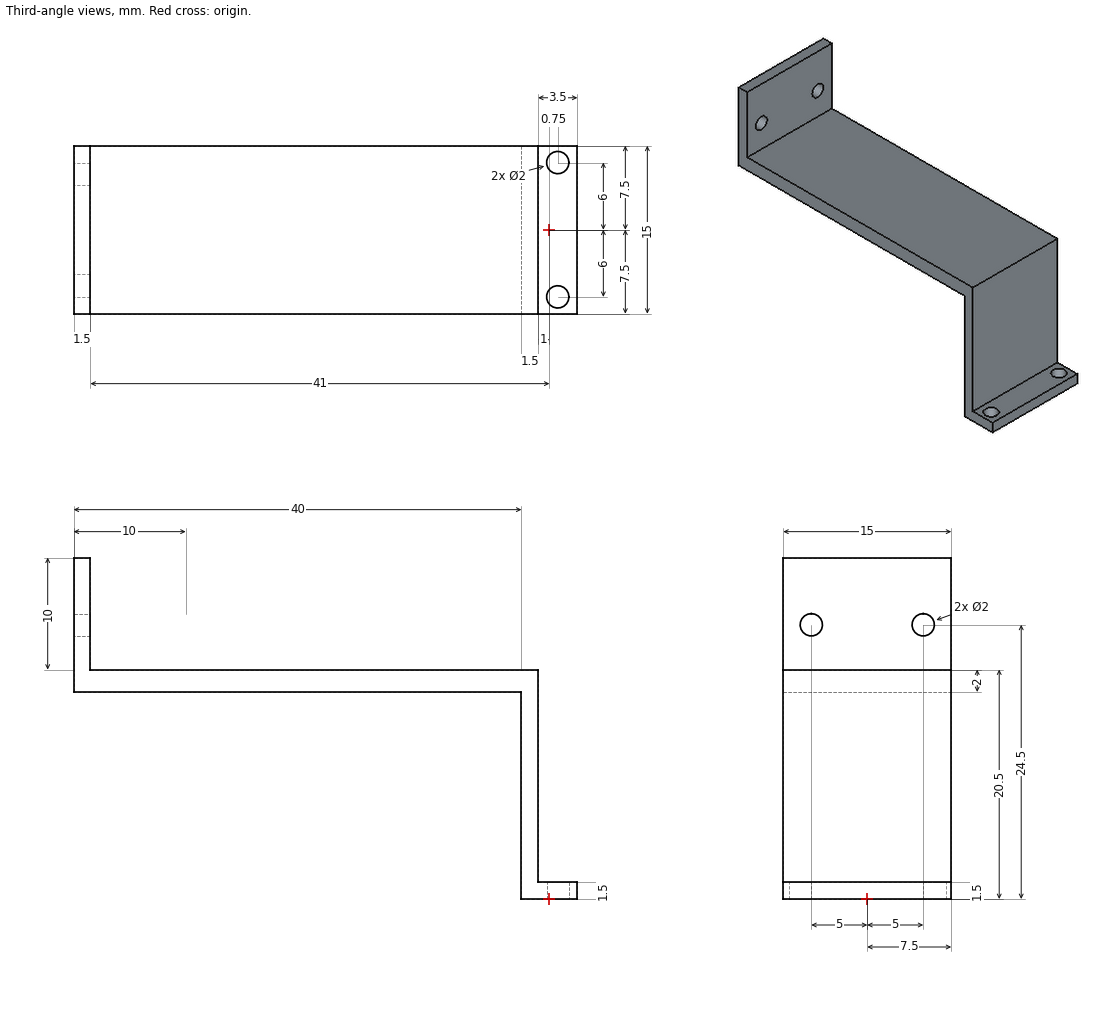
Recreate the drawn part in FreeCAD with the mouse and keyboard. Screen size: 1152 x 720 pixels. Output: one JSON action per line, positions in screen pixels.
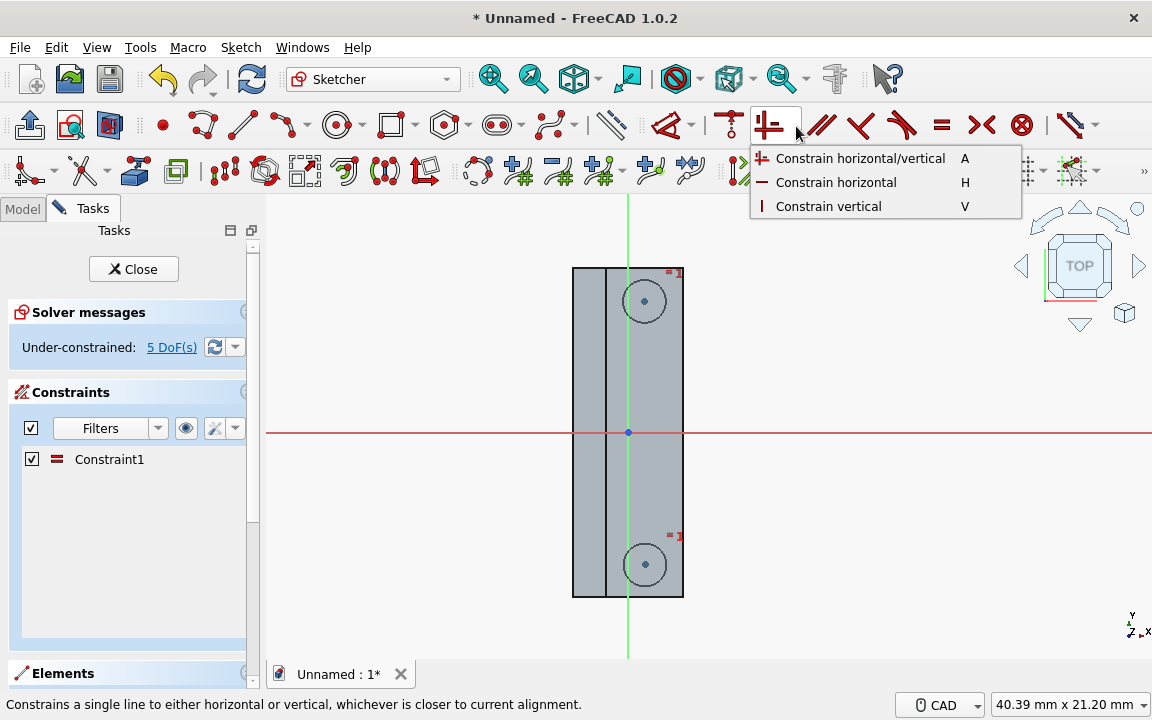
{"action": "left_click", "coordinate": [886, 206]}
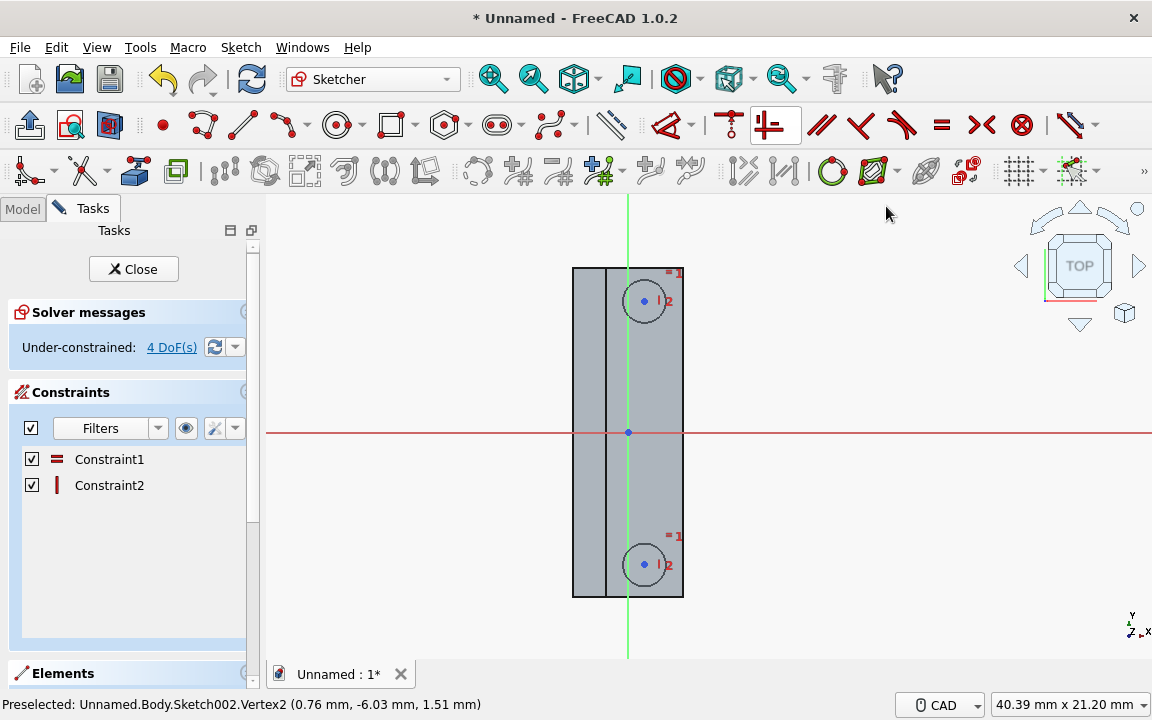
{"action": "left_click", "coordinate": [666, 126]}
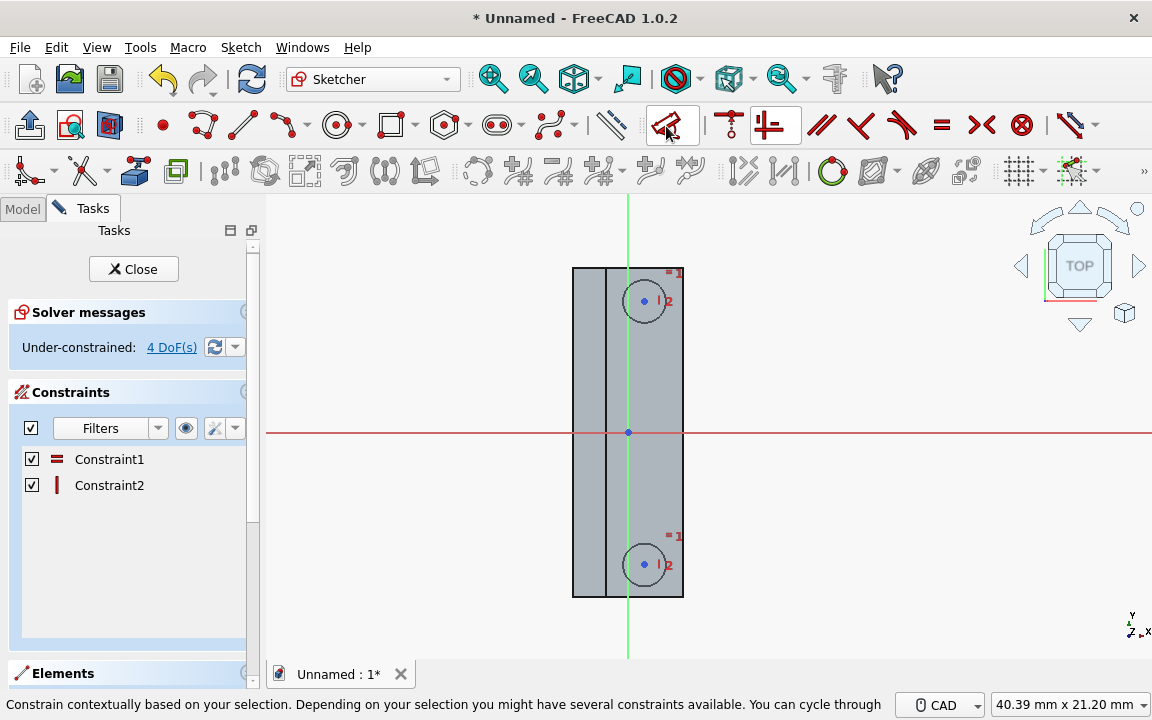
{"action": "left_click", "coordinate": [660, 286]}
{"action": "left_click", "coordinate": [683, 263]}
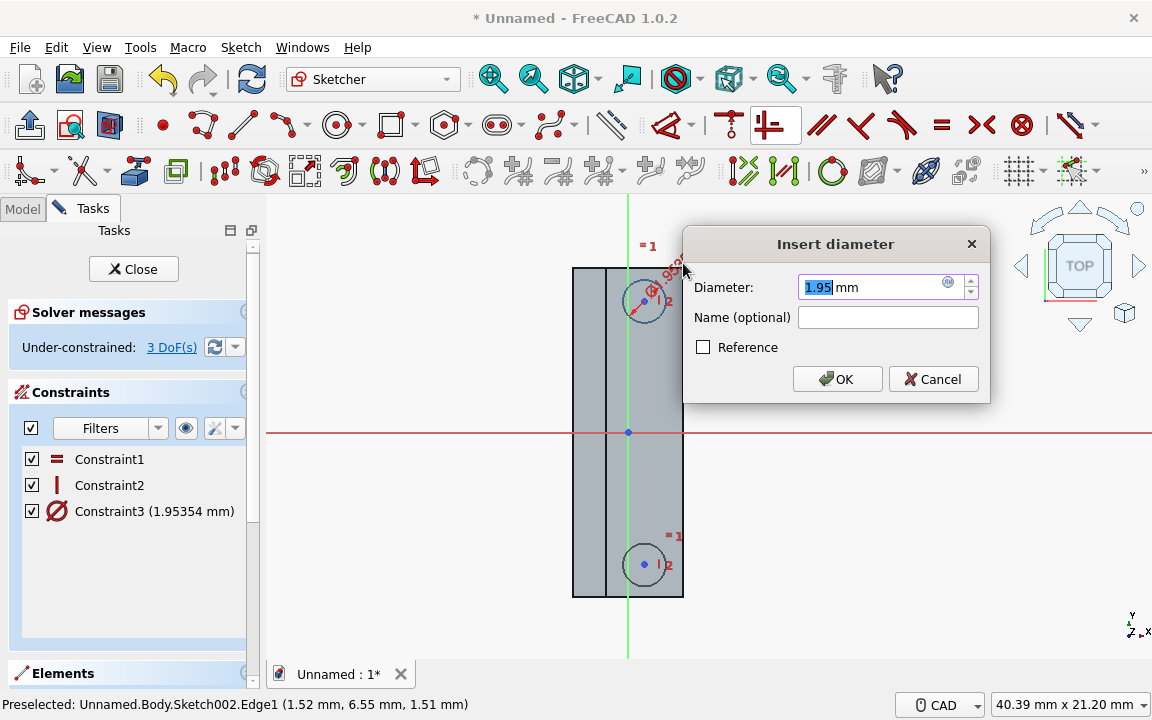
{"action": "type", "text": "2"}
{"action": "key", "text": "Return"}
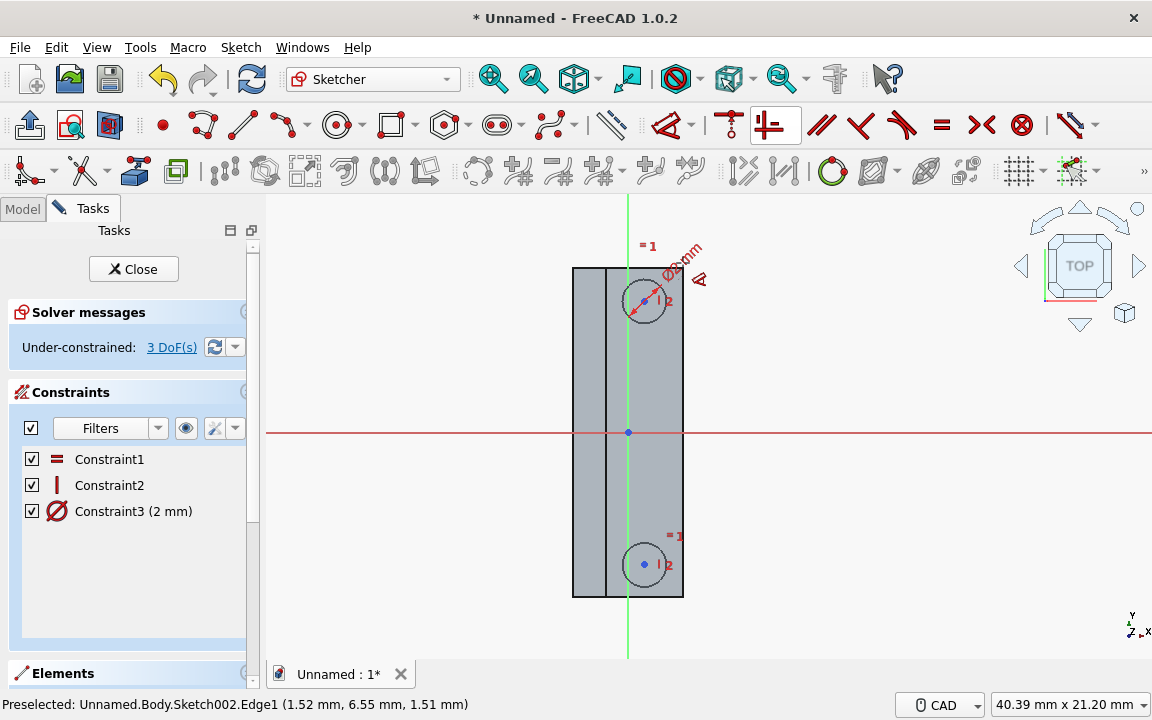
{"action": "left_click", "coordinate": [644, 301]}
{"action": "left_click", "coordinate": [594, 367]}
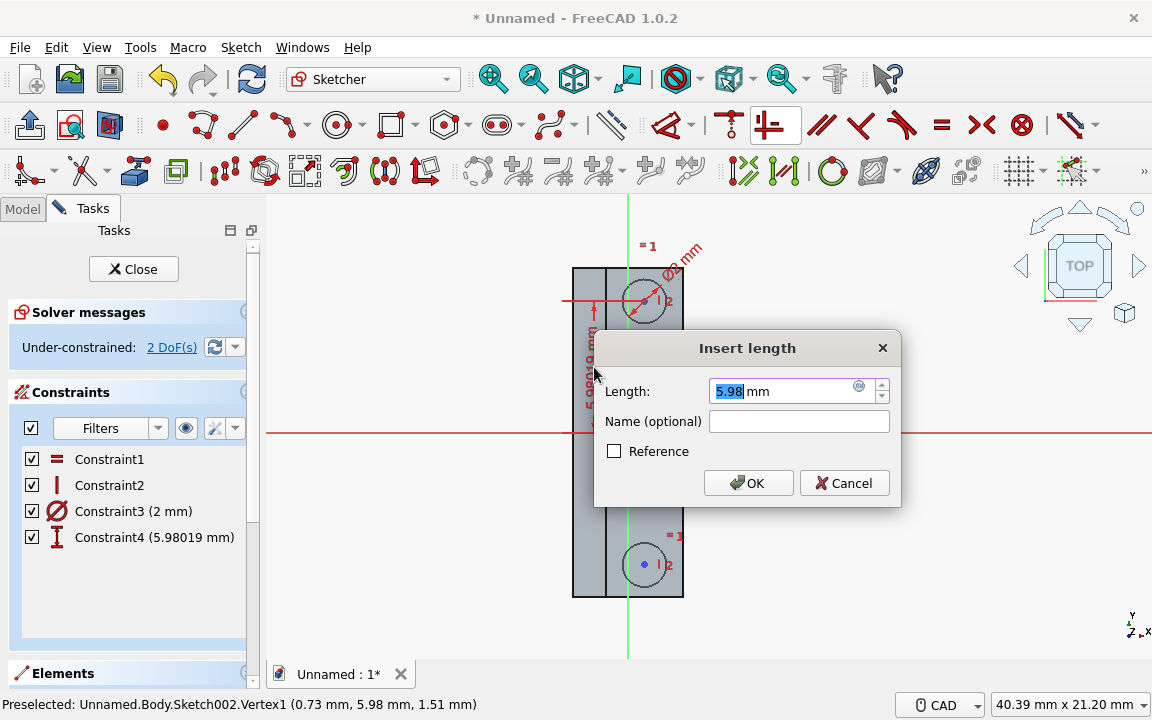
{"action": "type", "text": "6"}
{"action": "key", "text": "Return"}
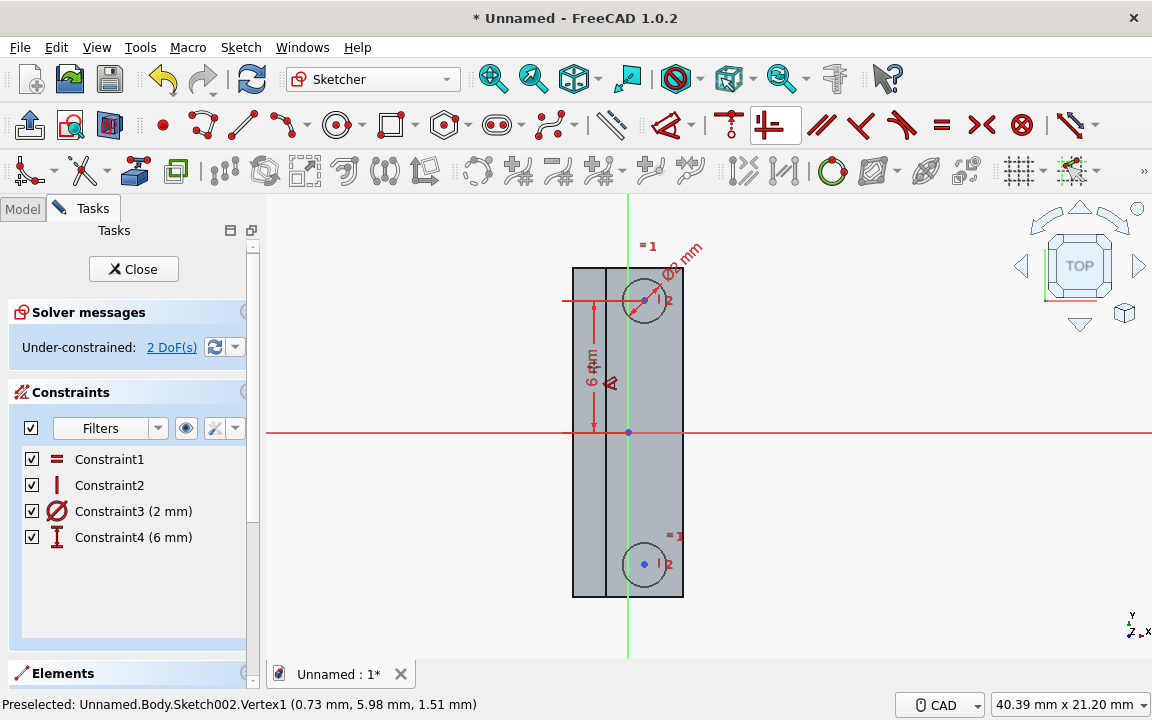
{"action": "left_click", "coordinate": [644, 565]}
{"action": "left_click", "coordinate": [594, 499]}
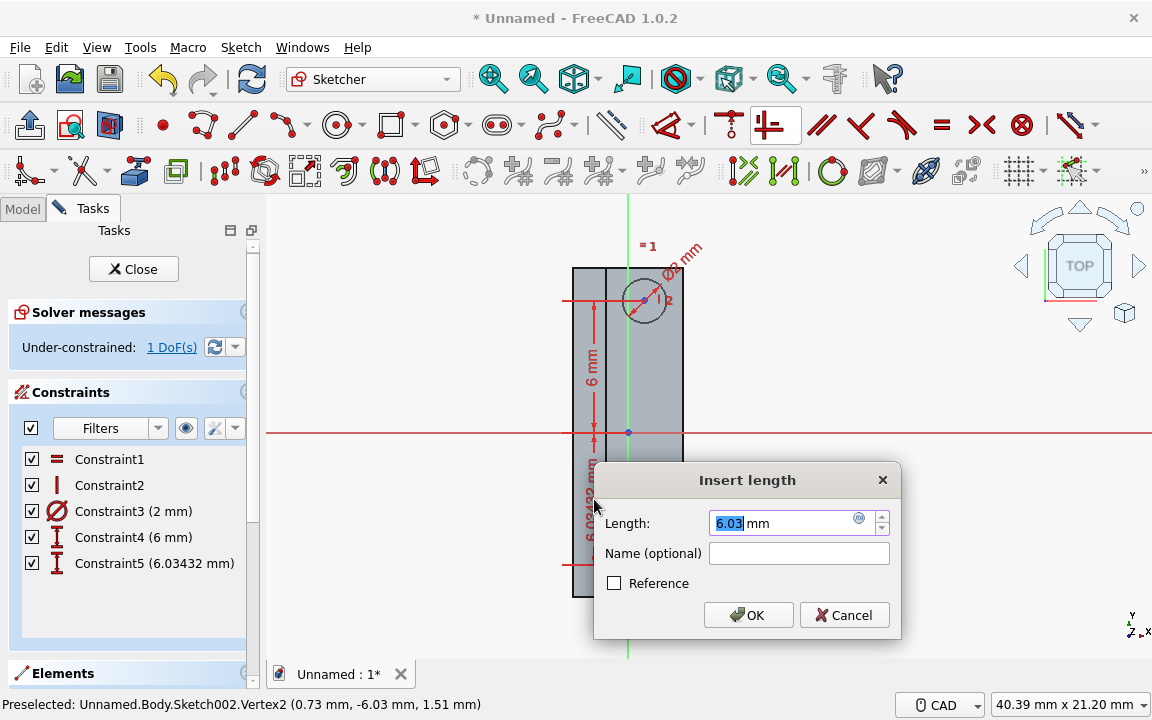
{"action": "type", "text": "6"}
{"action": "key", "text": "Return"}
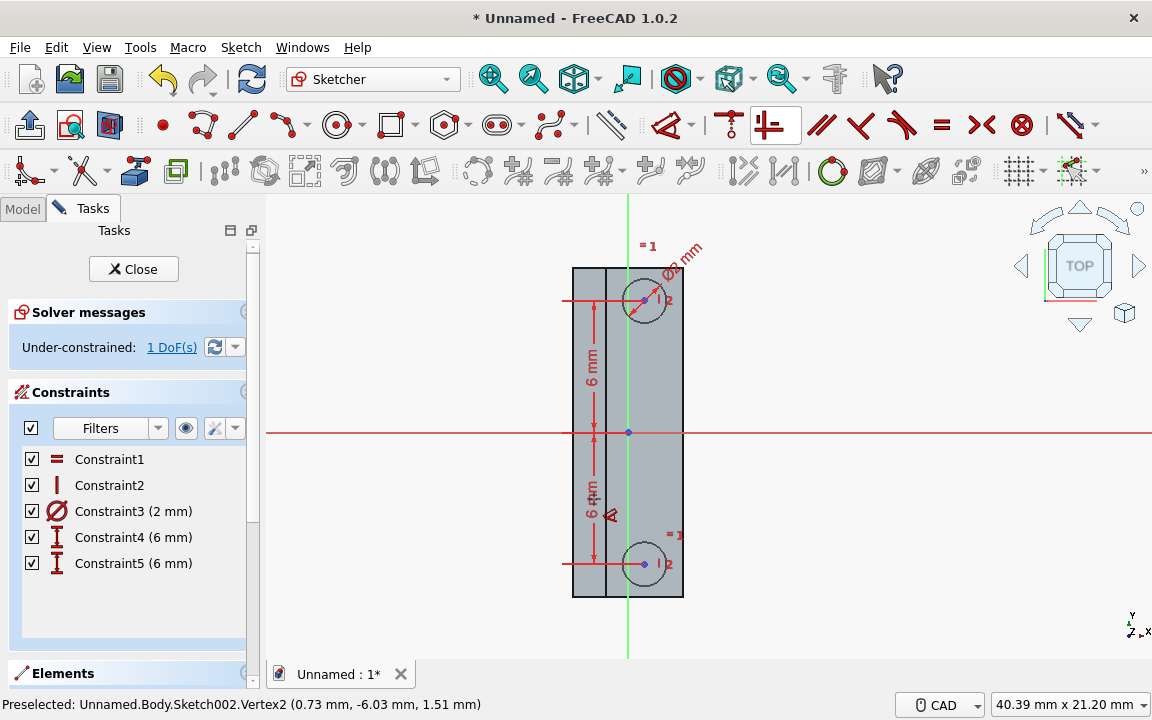
{"action": "scroll", "coordinate": [644, 301], "scroll_direction": "up", "scroll_amount": 5}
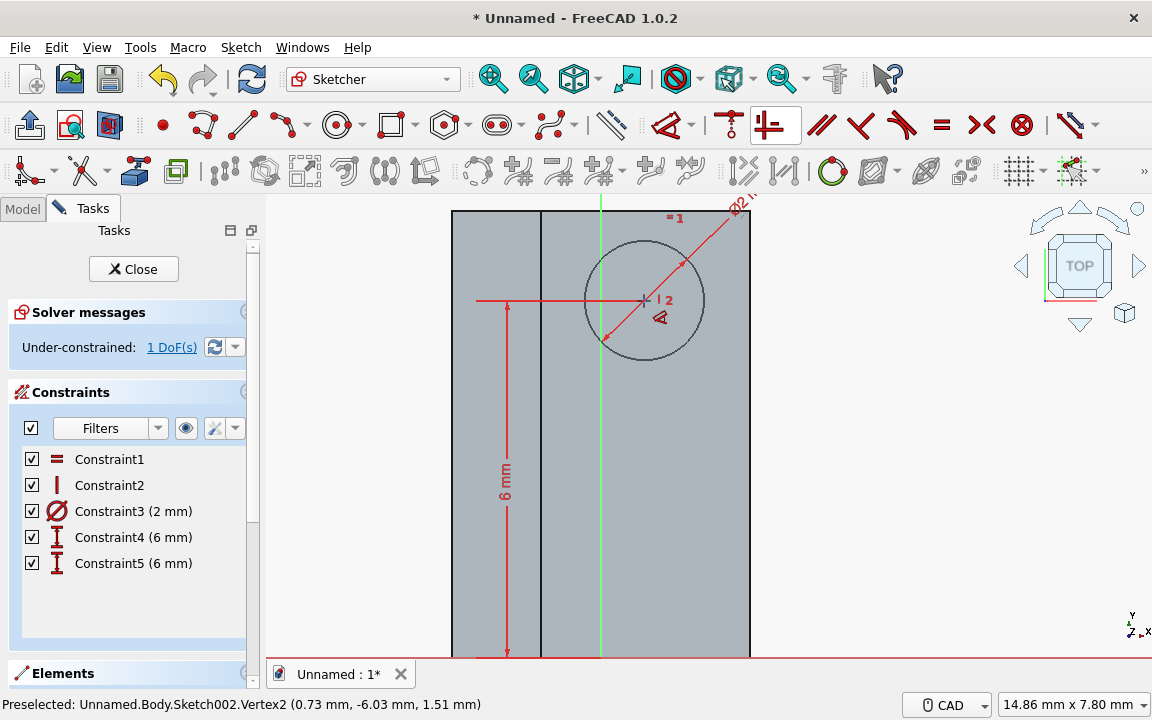
{"action": "left_click", "coordinate": [644, 301]}
{"action": "left_click", "coordinate": [623, 267]}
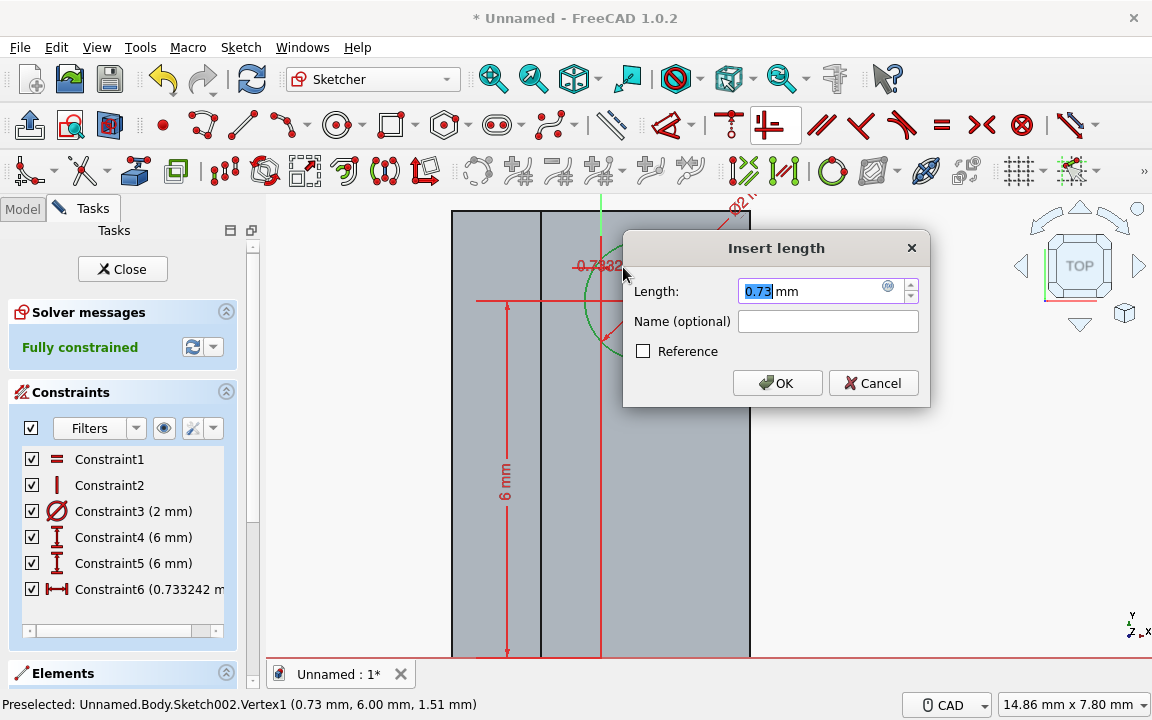
{"action": "type", "text": "0.75"}
{"action": "key", "text": "Return"}
{"action": "key", "text": "Escape"}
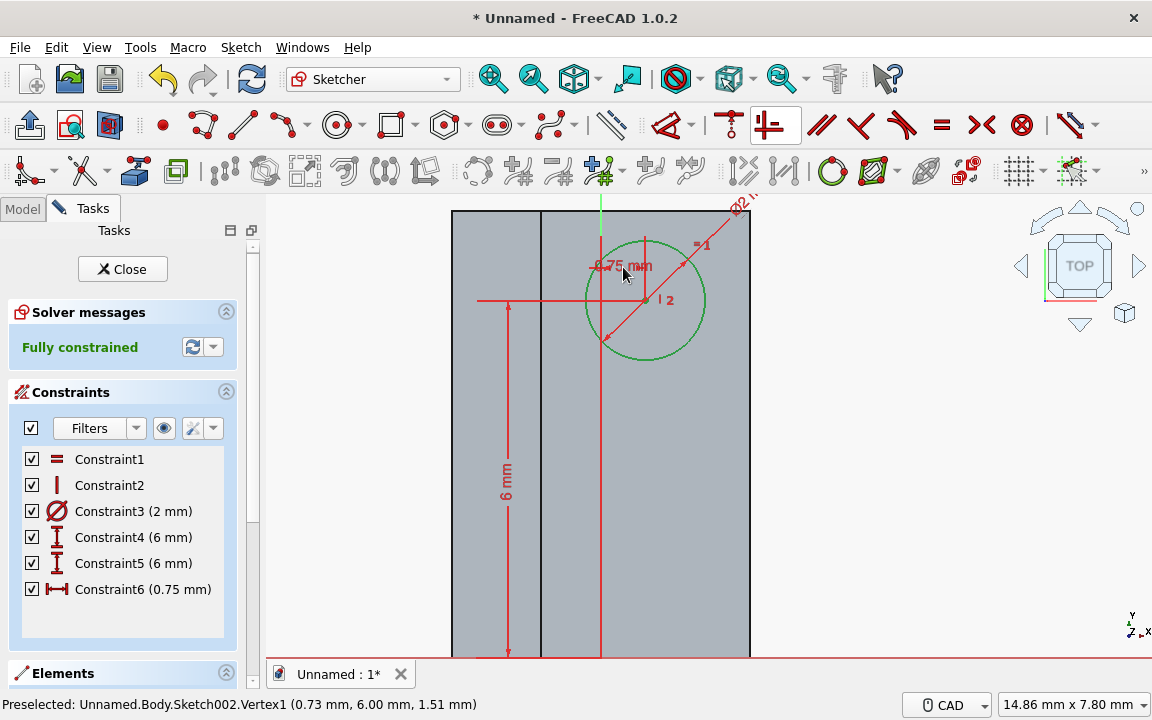
{"action": "left_click", "coordinate": [123, 269]}